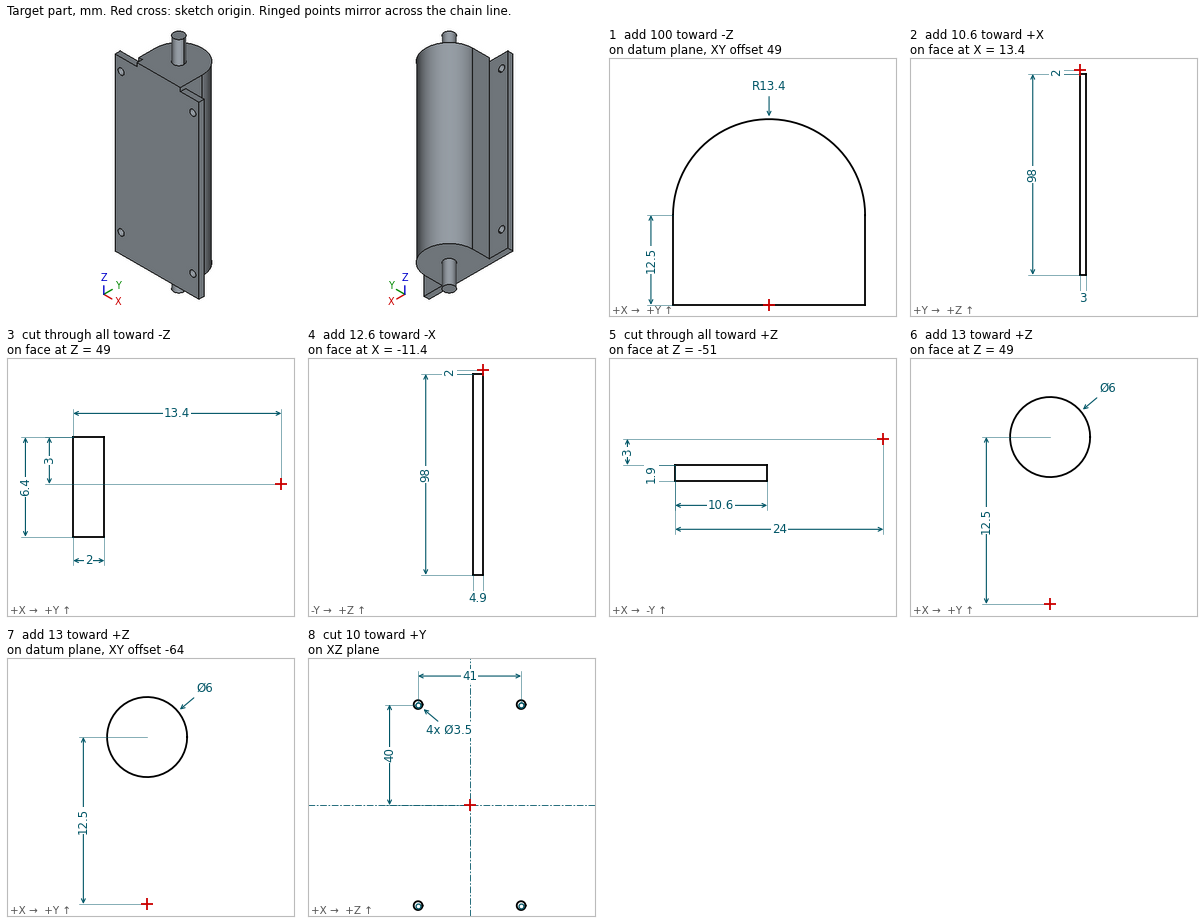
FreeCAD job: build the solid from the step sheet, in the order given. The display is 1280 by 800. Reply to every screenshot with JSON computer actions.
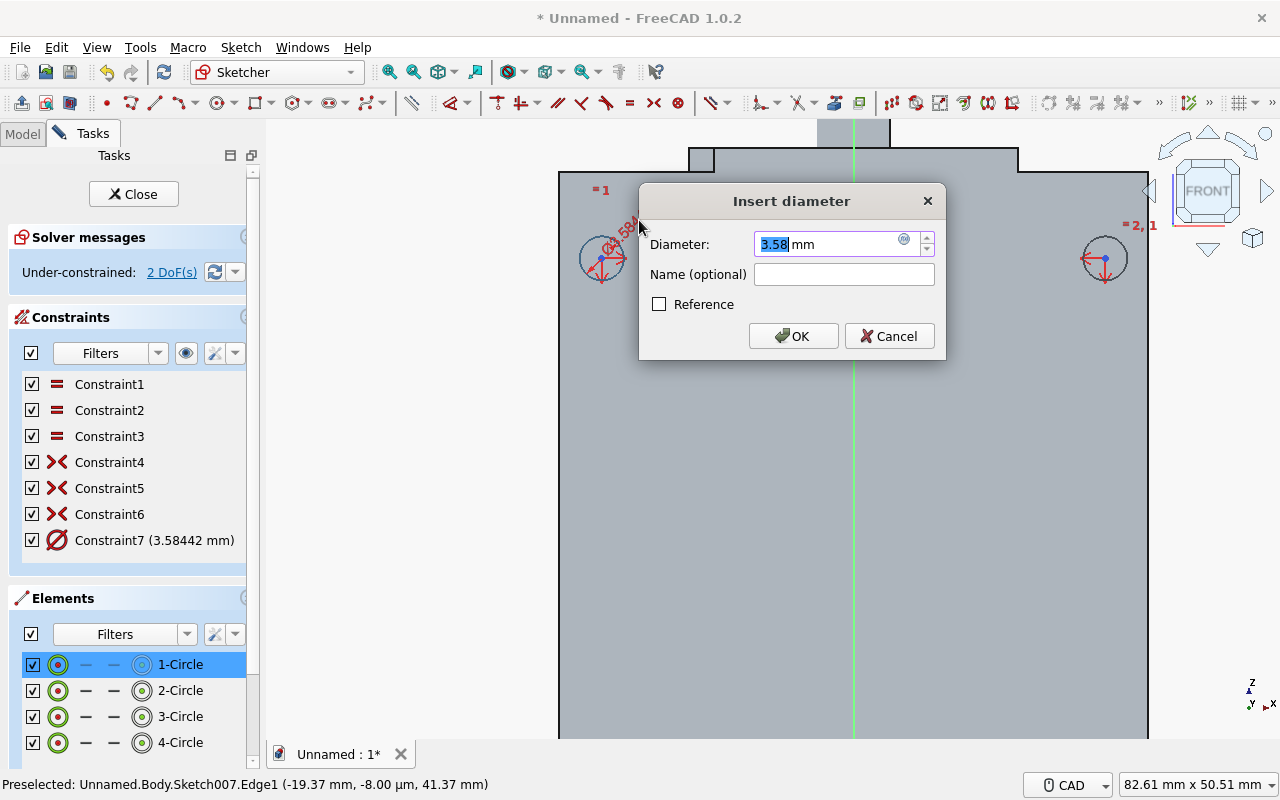
{"action": "type", "text": "3.5"}
{"action": "key", "text": "Return"}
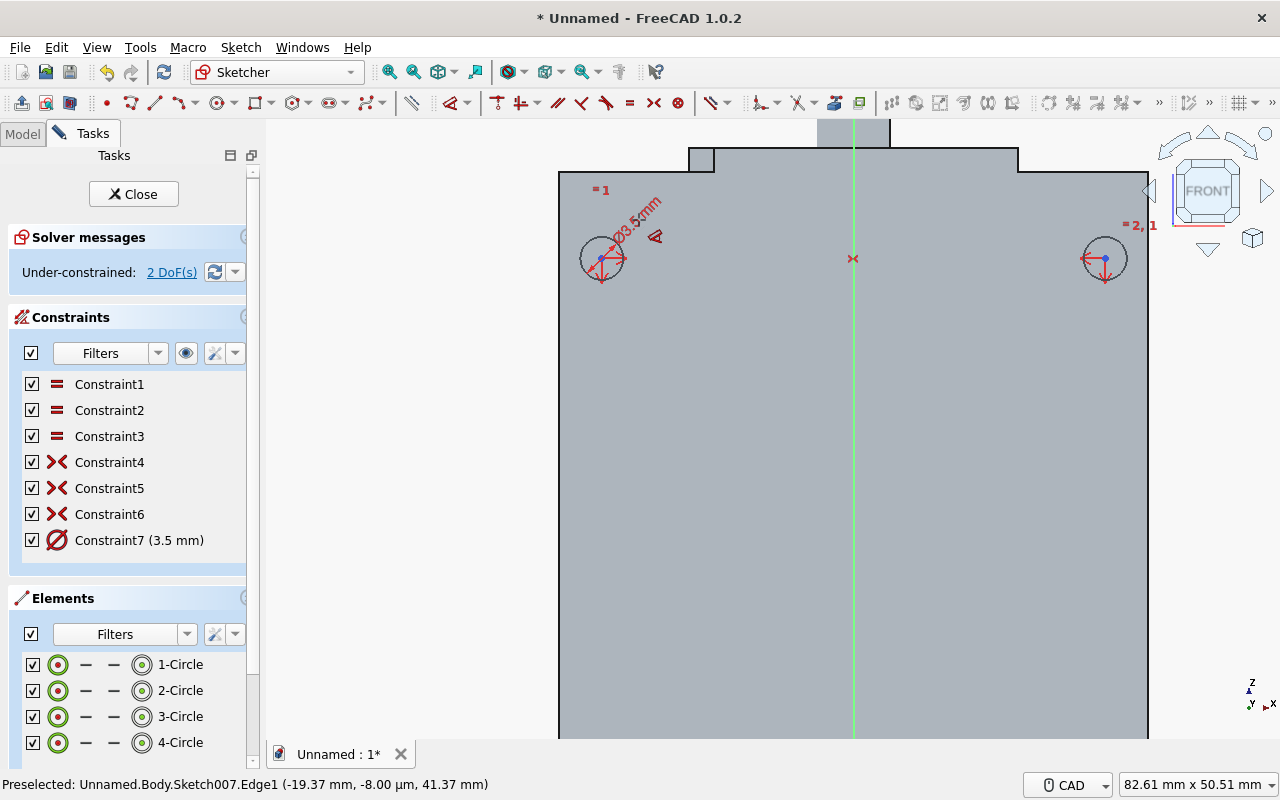
{"action": "left_click", "coordinate": [602, 258]}
{"action": "left_click", "coordinate": [568, 485]}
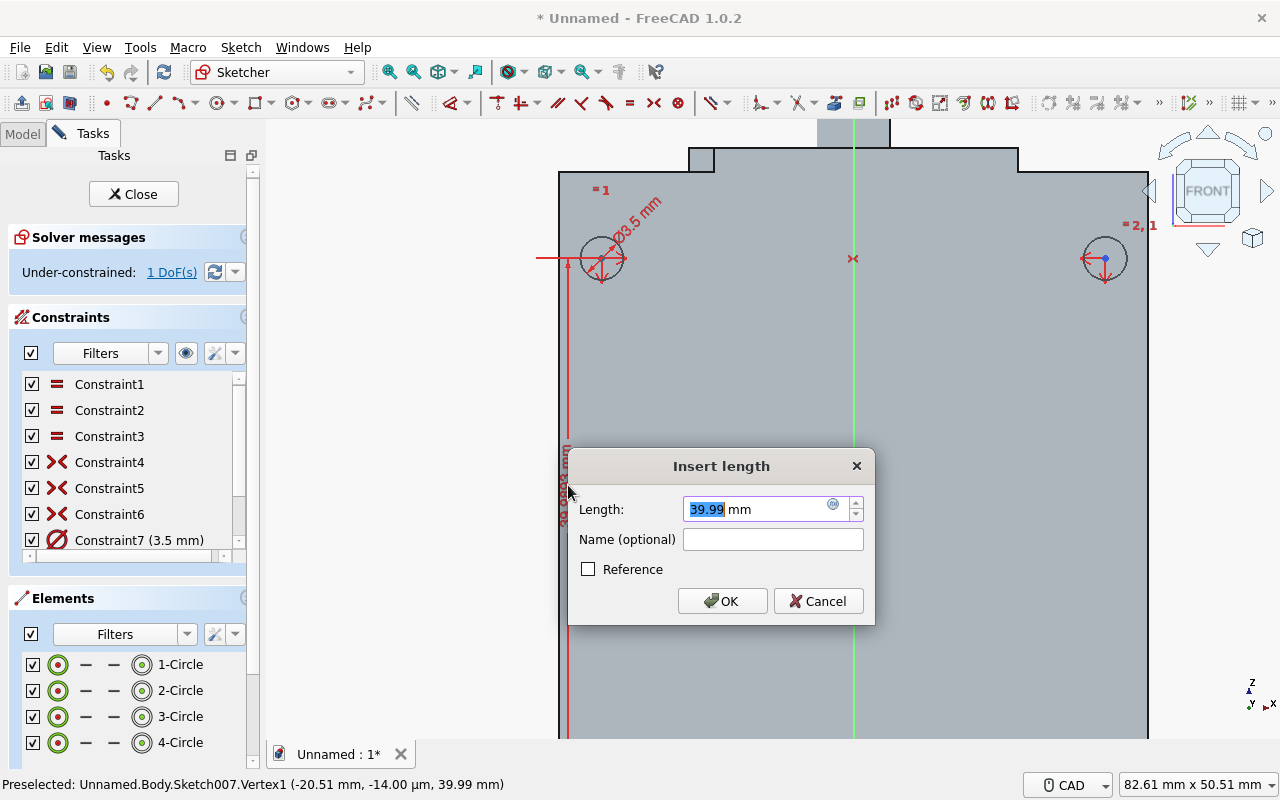
{"action": "type", "text": "40"}
{"action": "key", "text": "Return"}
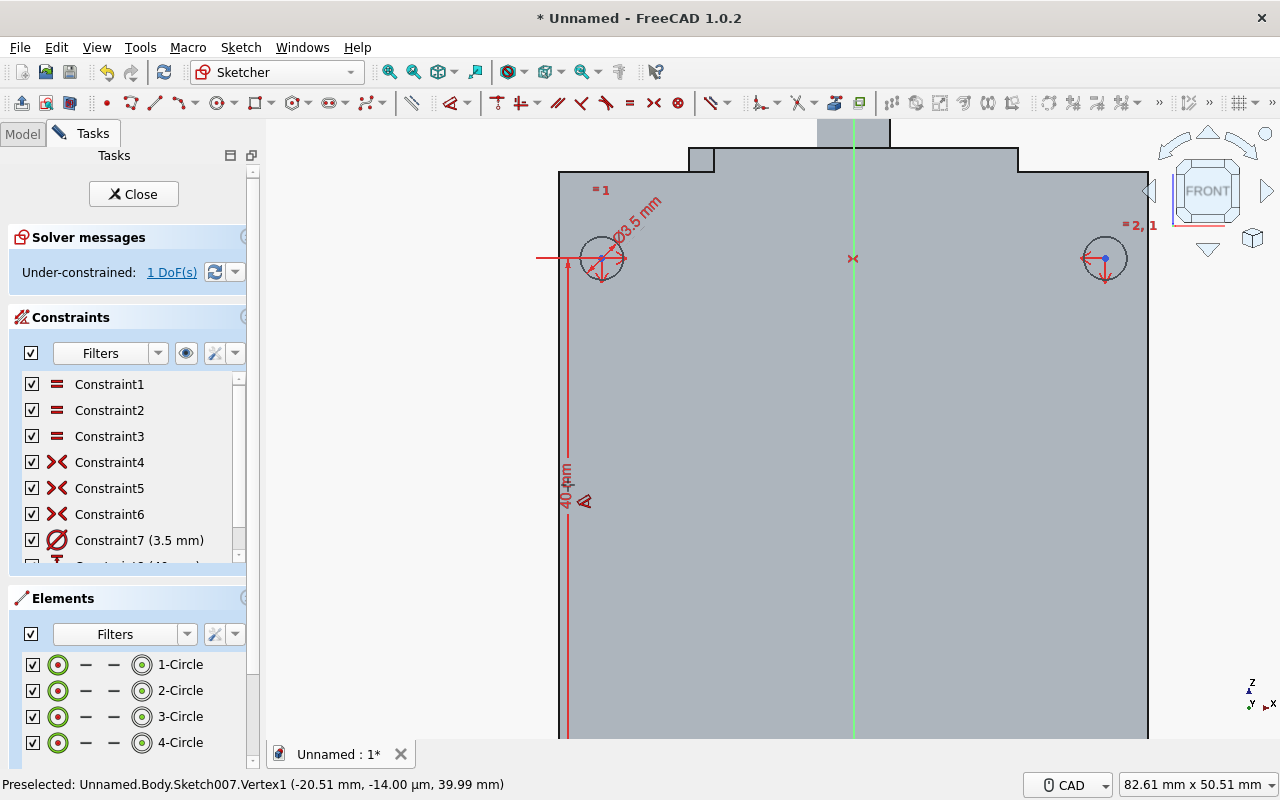
{"action": "left_click", "coordinate": [602, 258]}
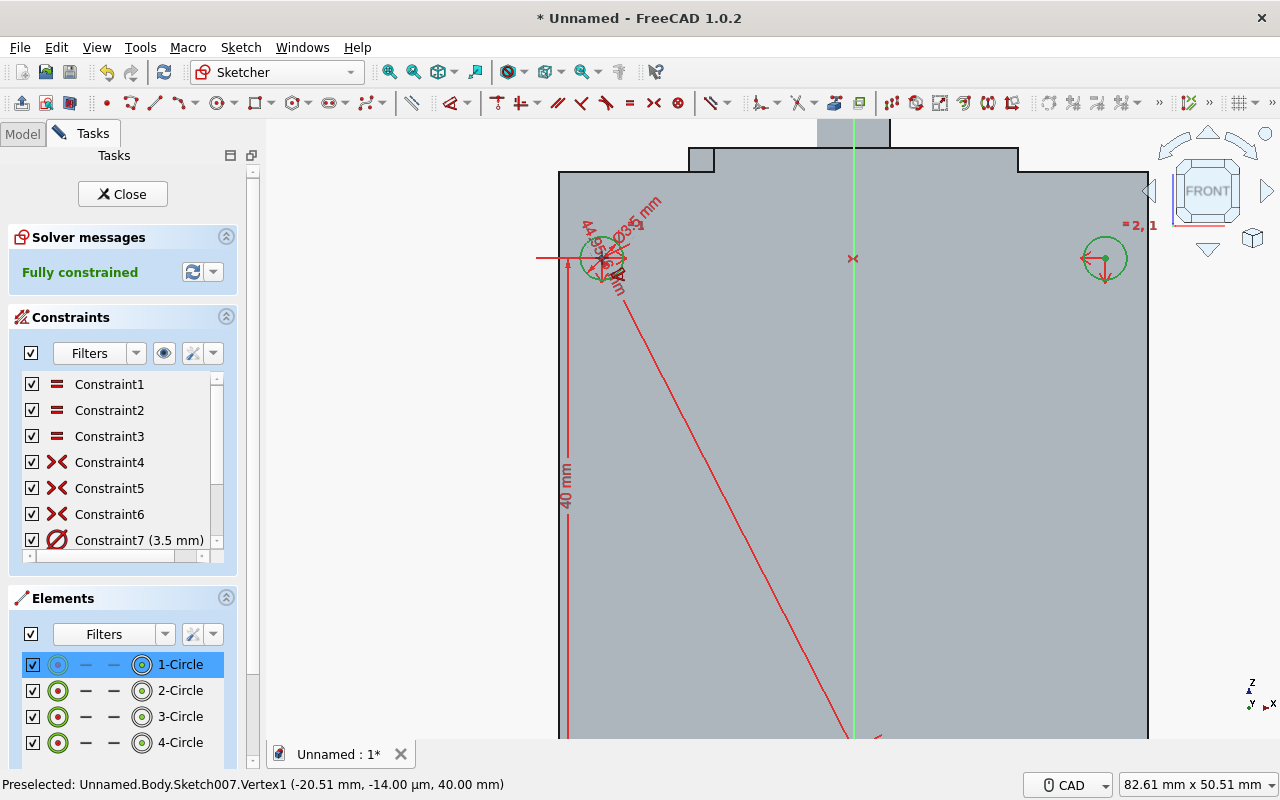
{"action": "left_click", "coordinate": [1105, 258]}
{"action": "left_click", "coordinate": [738, 224]}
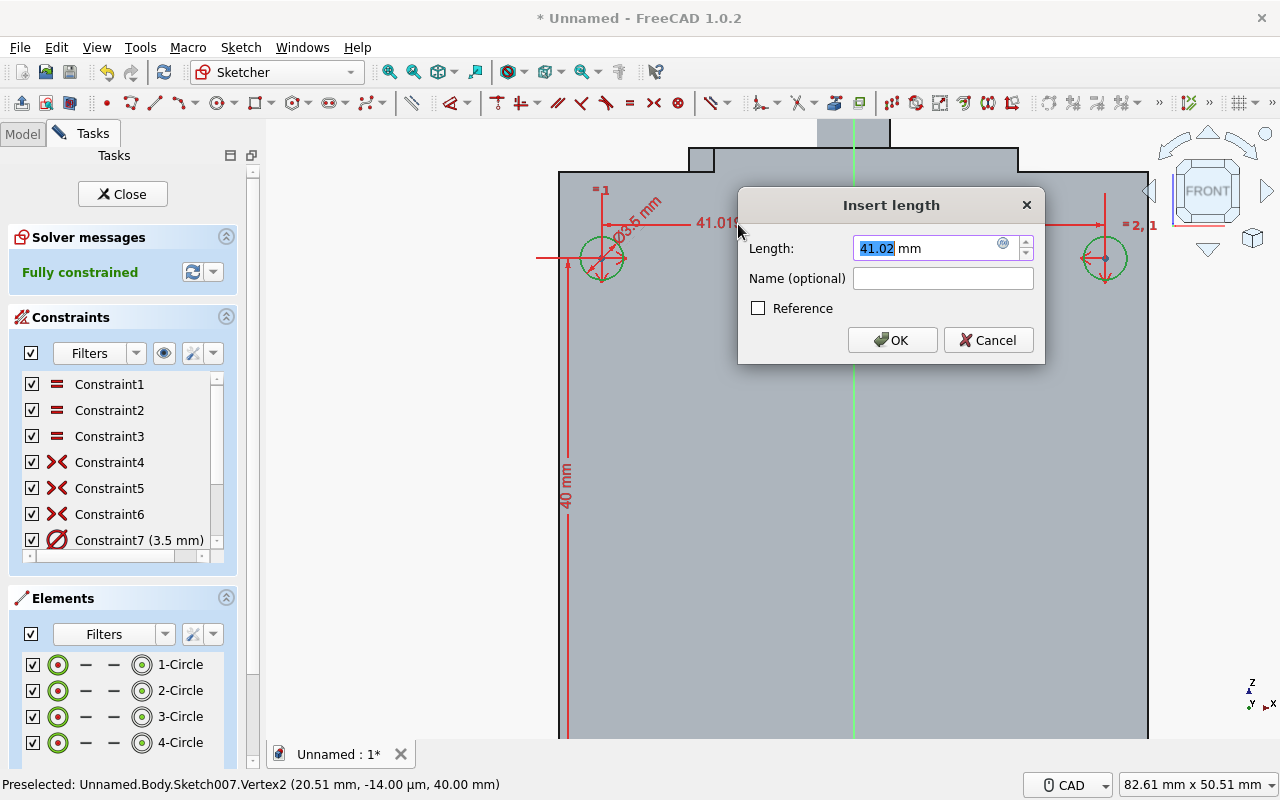
{"action": "type", "text": "41"}
{"action": "key", "text": "Return"}
{"action": "key", "text": "Escape"}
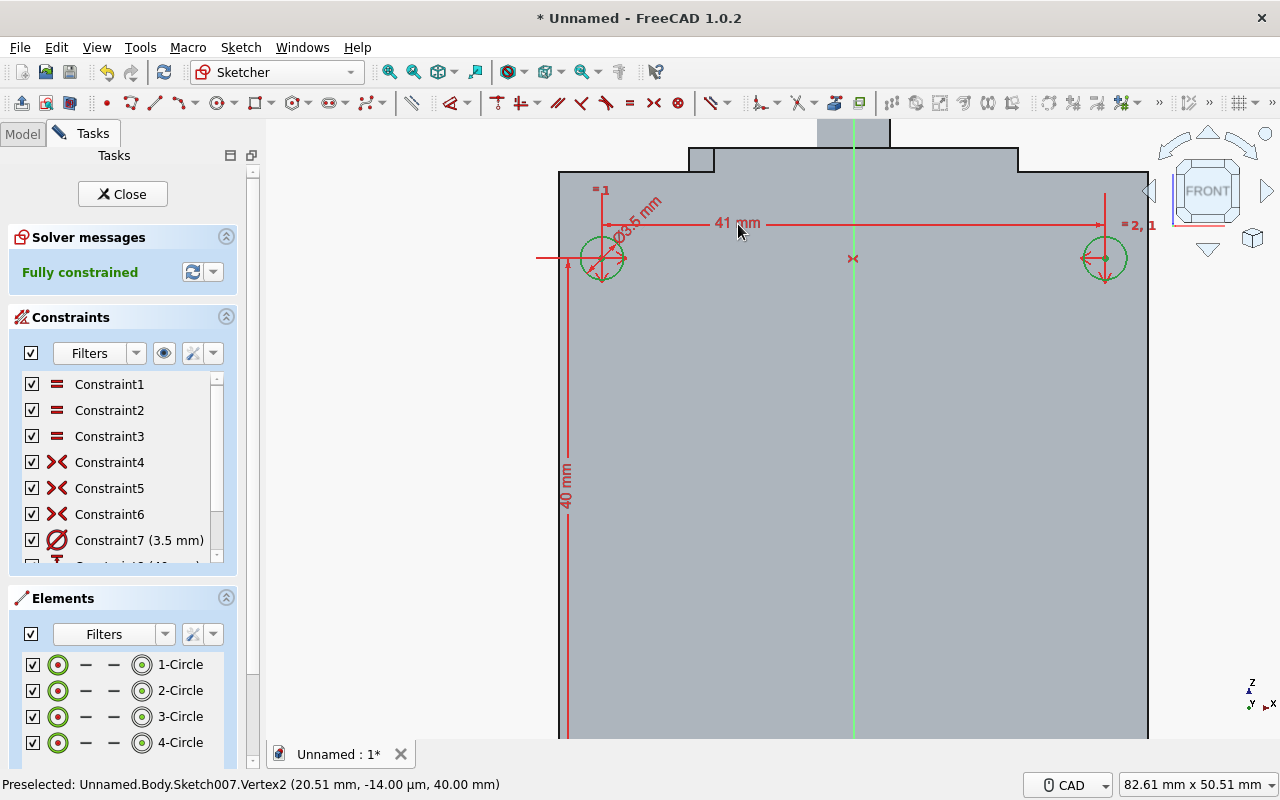
{"action": "left_click", "coordinate": [123, 194]}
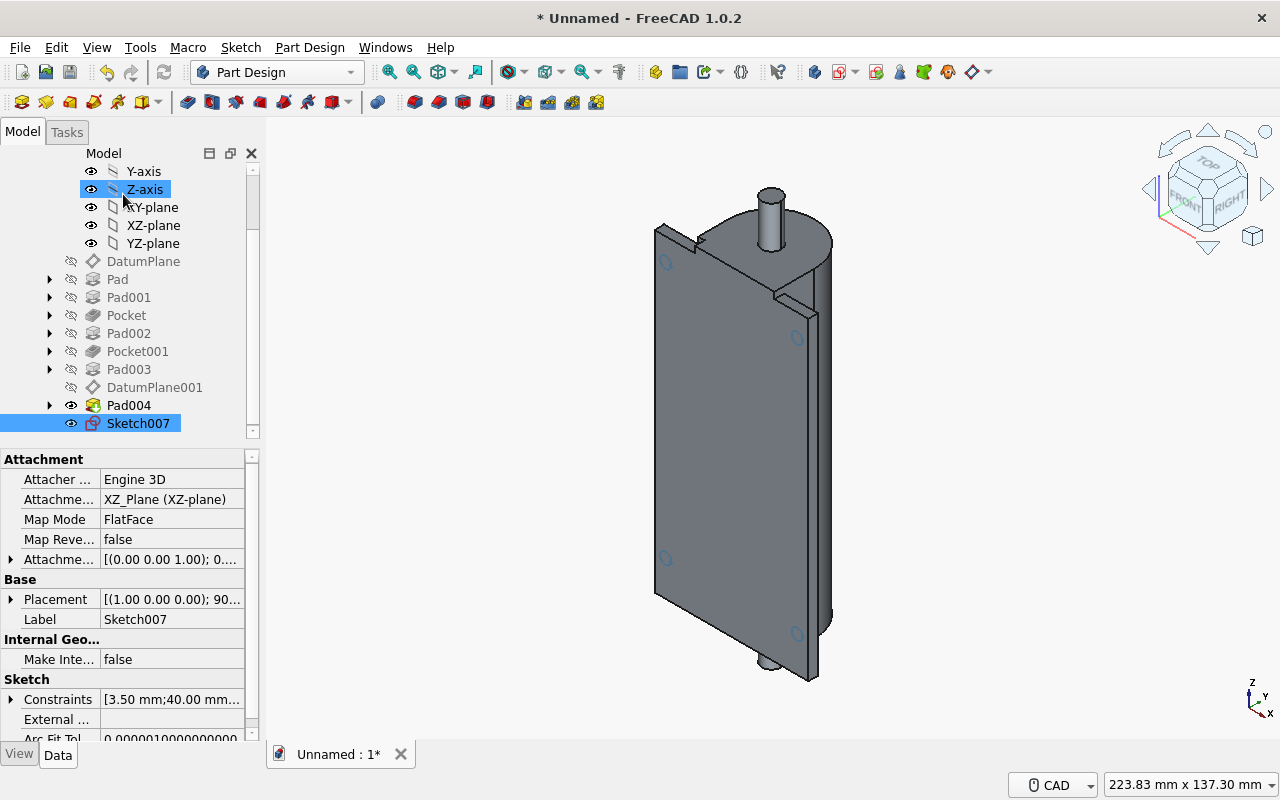
{"action": "left_click", "coordinate": [188, 102]}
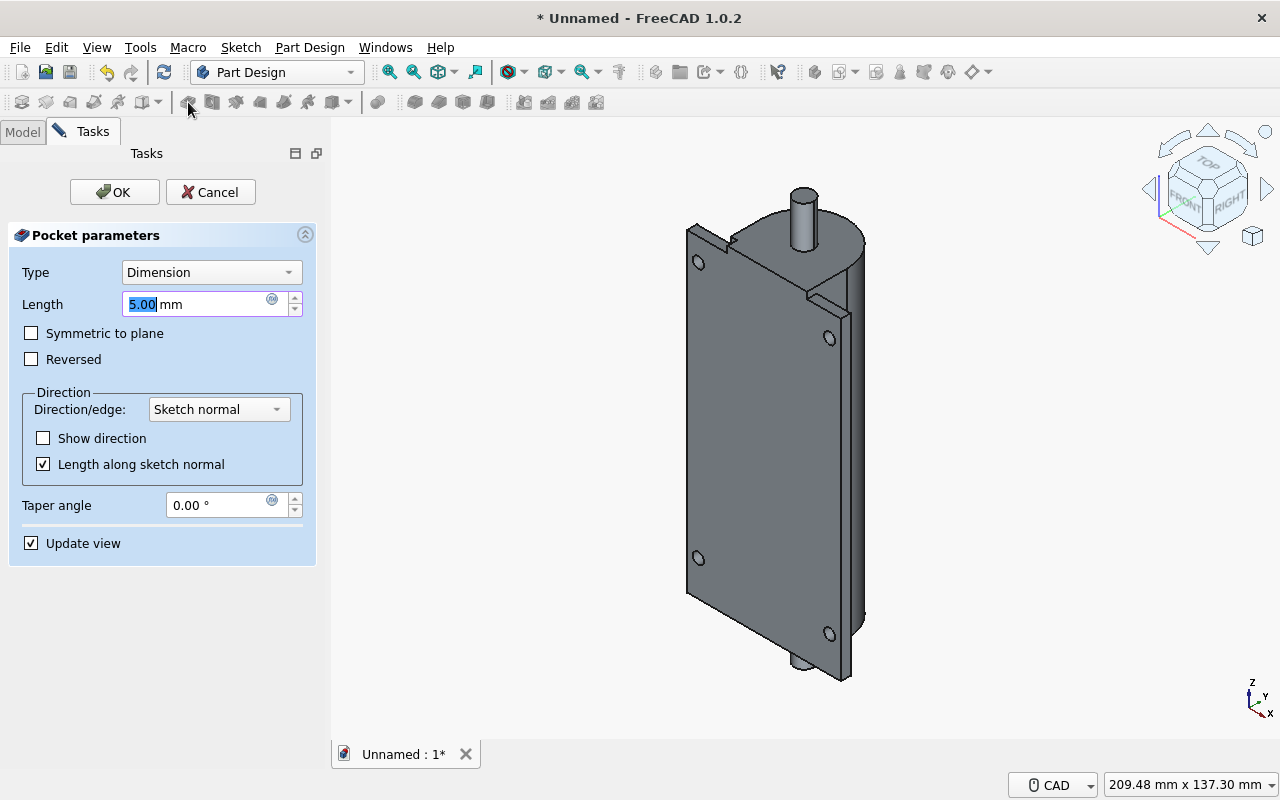
{"action": "type", "text": "10"}
{"action": "key", "text": "Tab"}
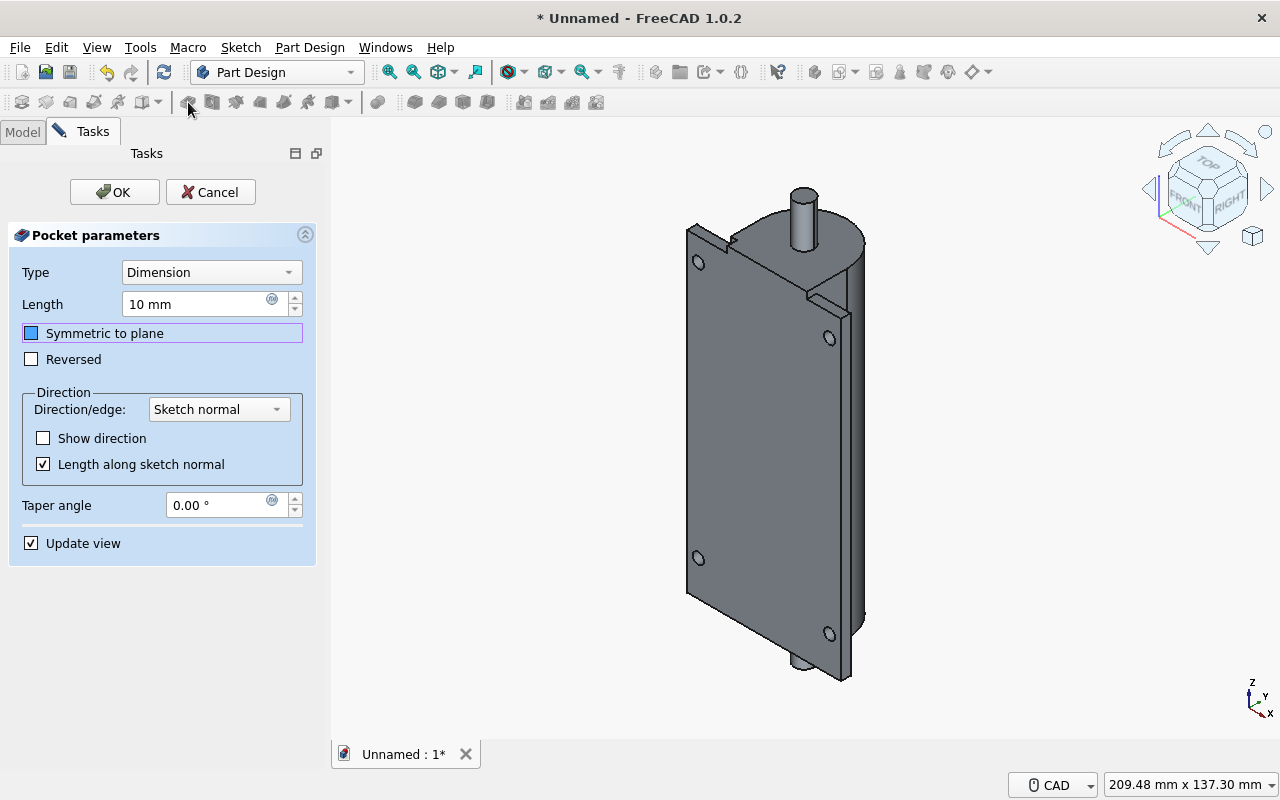
{"action": "left_click", "coordinate": [115, 192]}